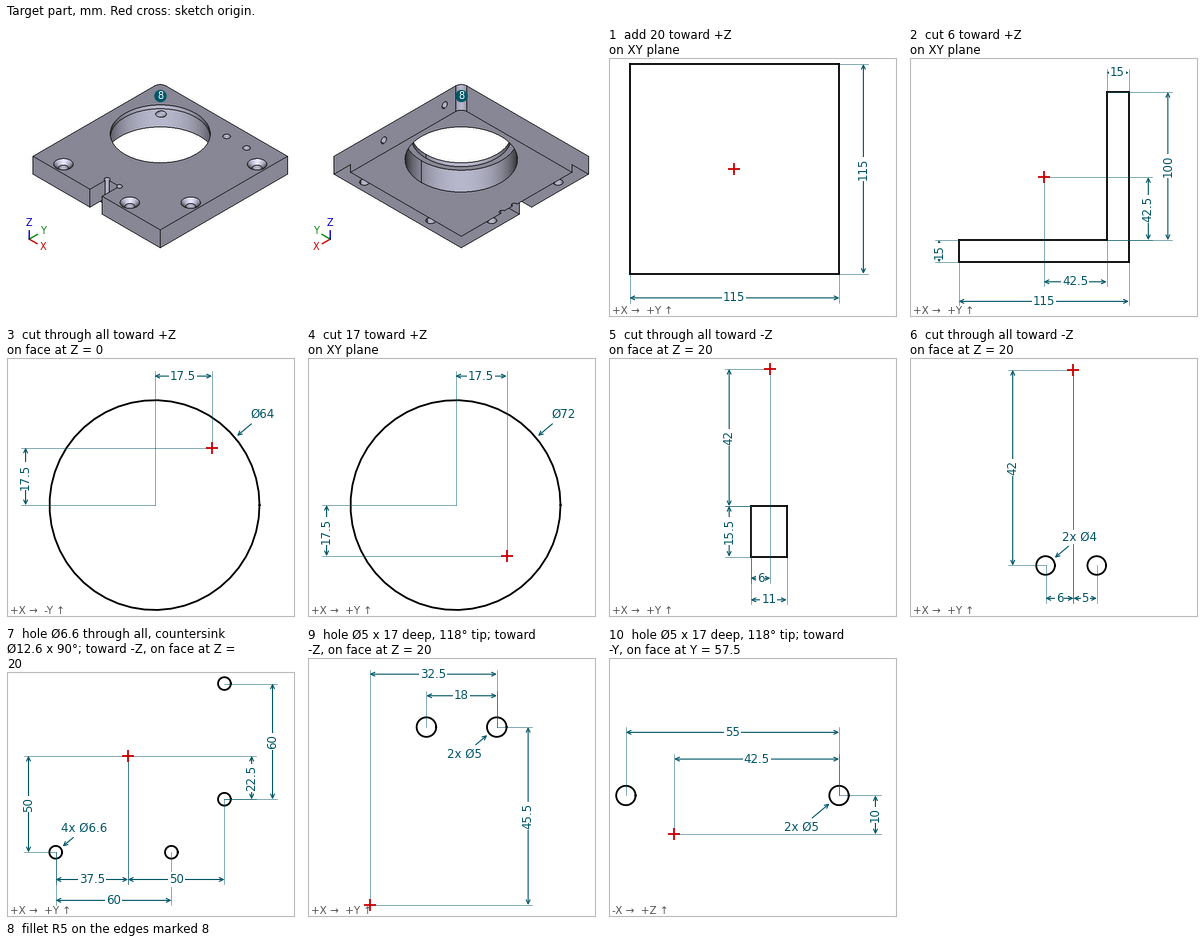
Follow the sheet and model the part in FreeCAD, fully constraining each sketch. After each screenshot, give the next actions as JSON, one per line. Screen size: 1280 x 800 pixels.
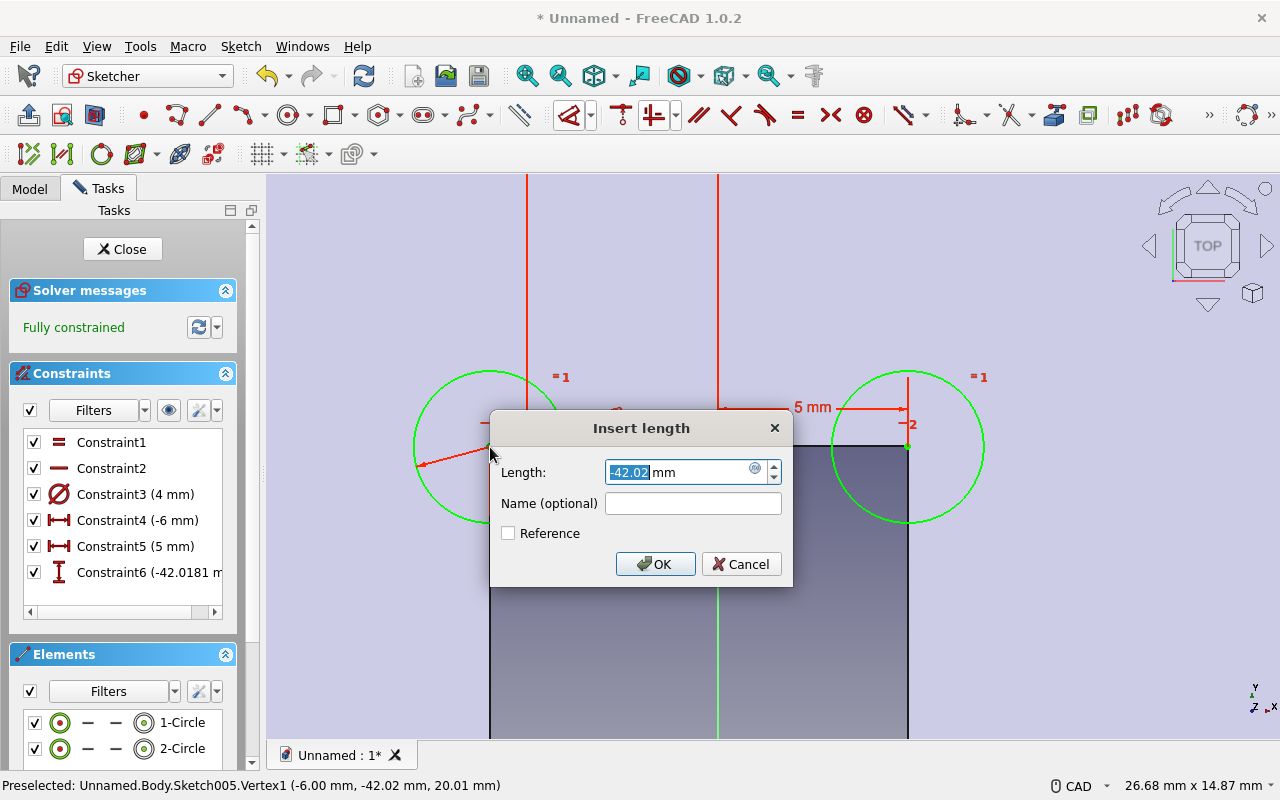
{"action": "type", "text": "-42"}
{"action": "key", "text": "Return"}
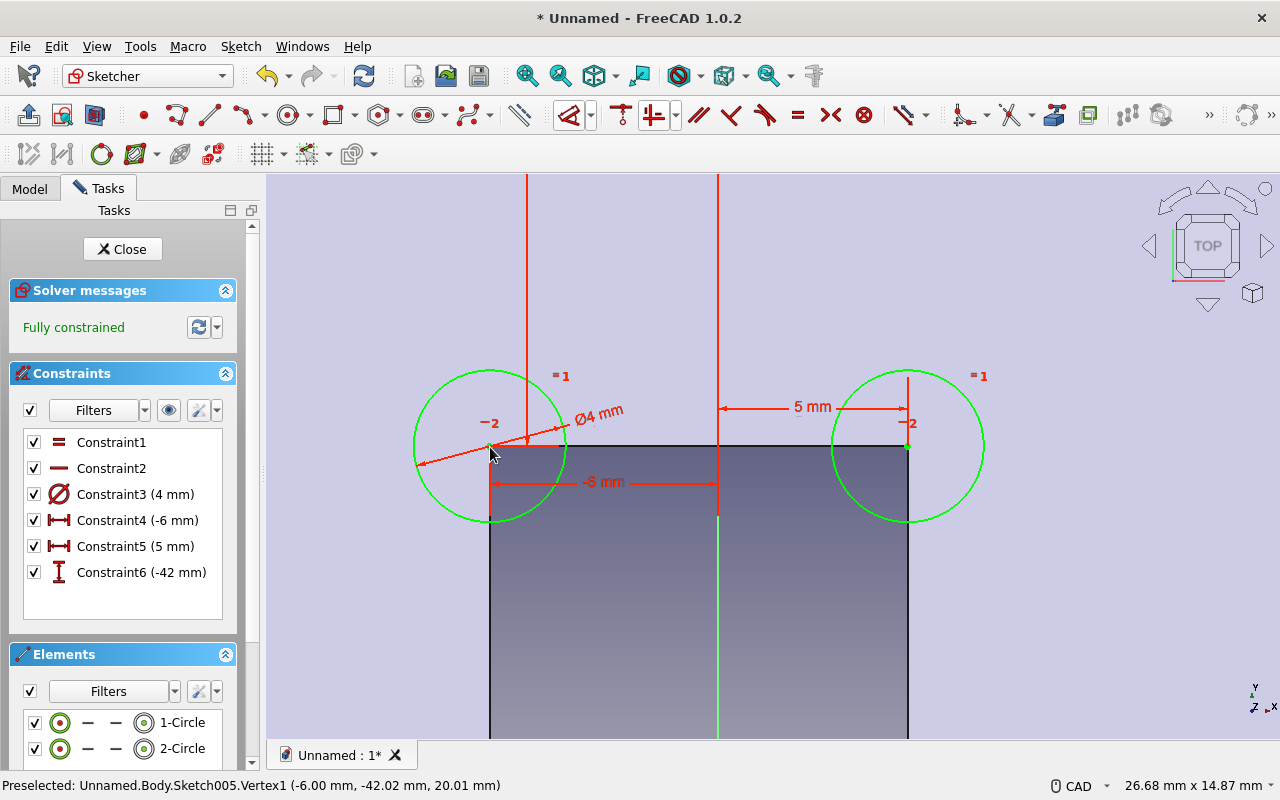
{"action": "left_click", "coordinate": [123, 249]}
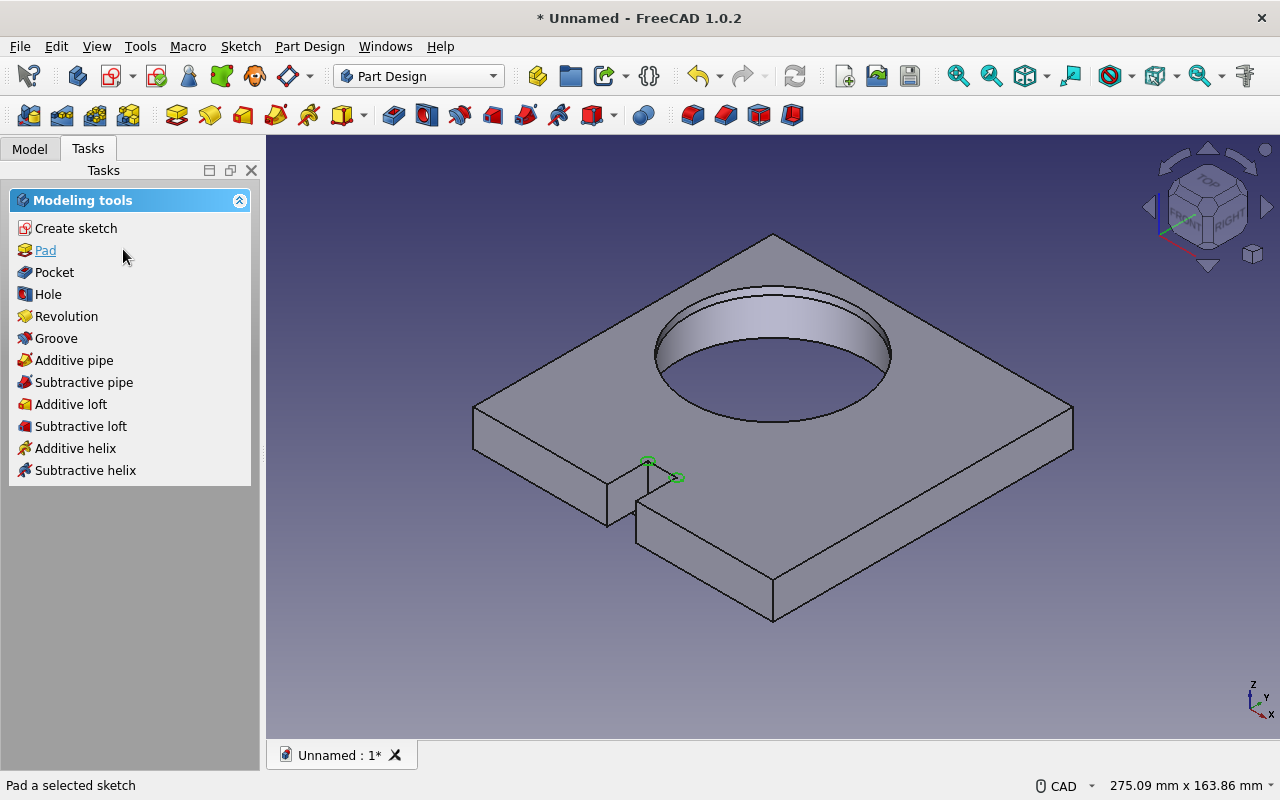
{"action": "left_click", "coordinate": [394, 116]}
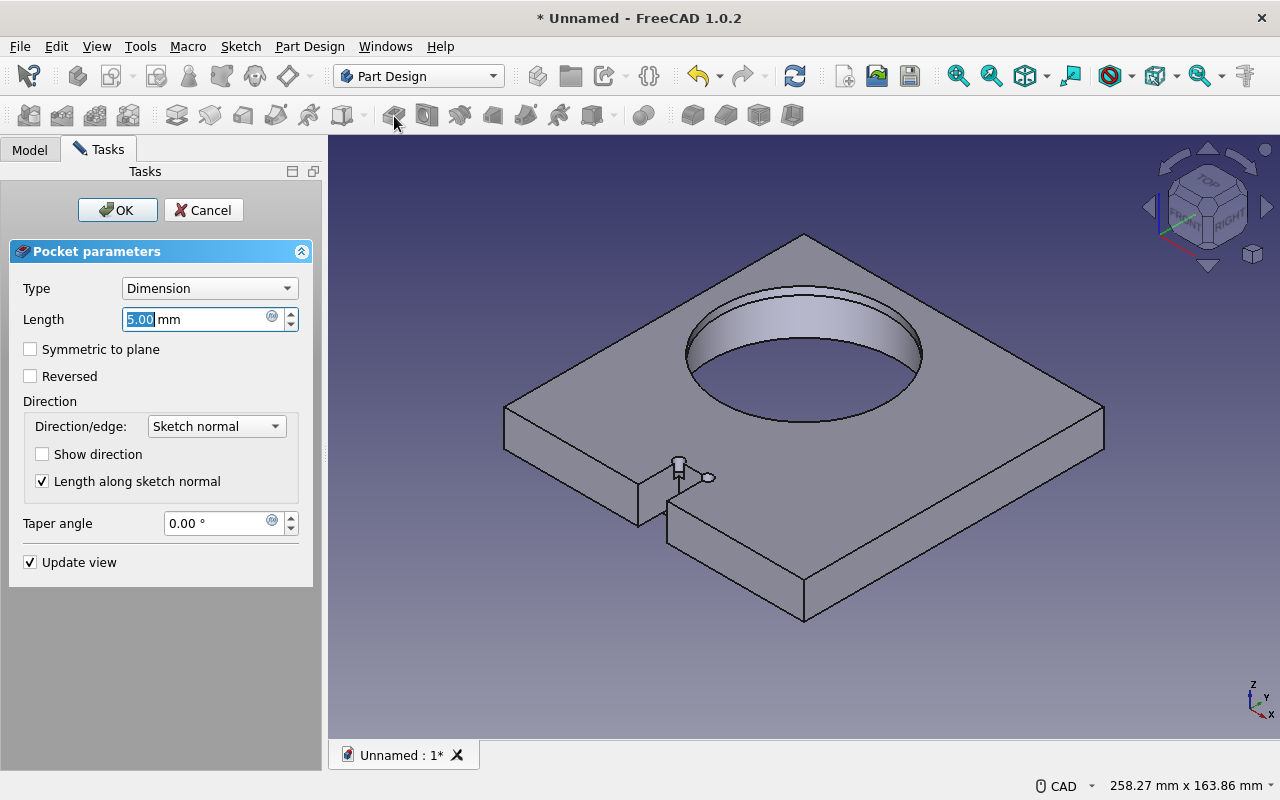
{"action": "left_click", "coordinate": [210, 288]}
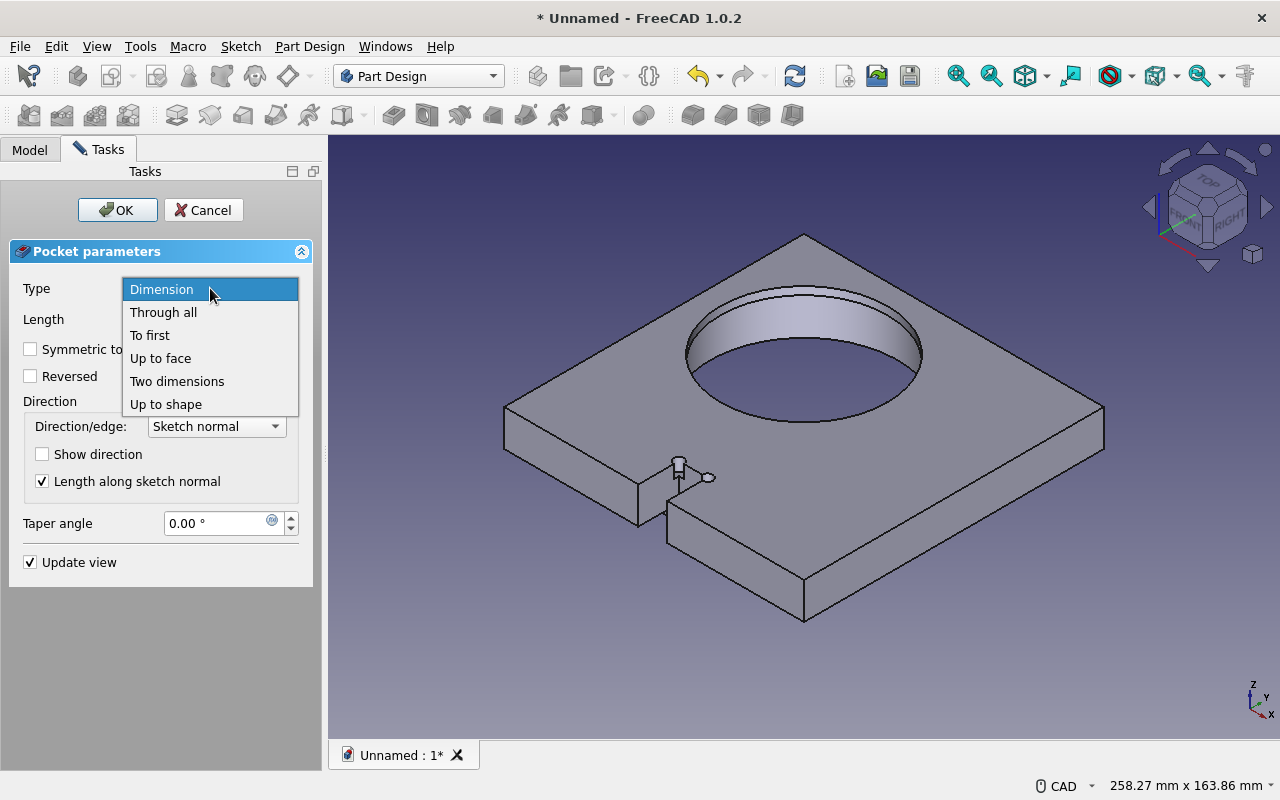
{"action": "left_click", "coordinate": [208, 312]}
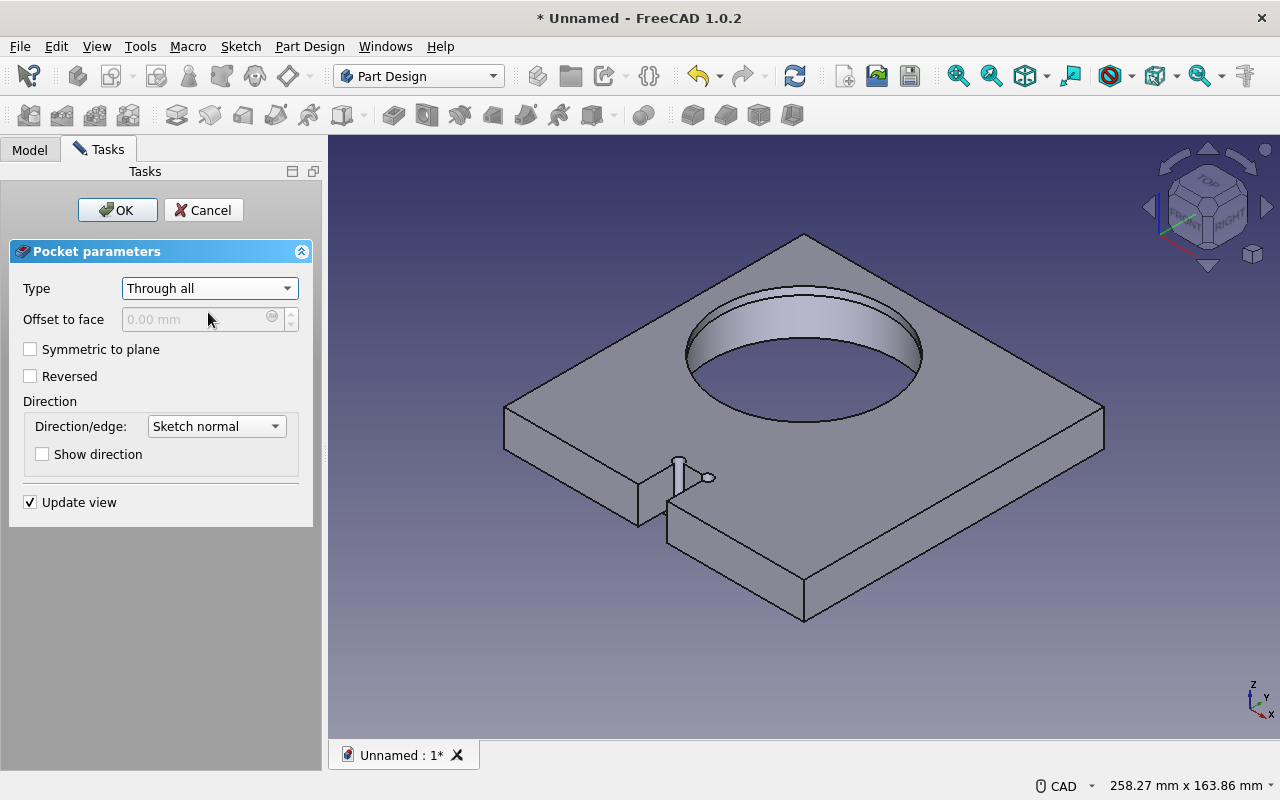
{"action": "left_click", "coordinate": [118, 210]}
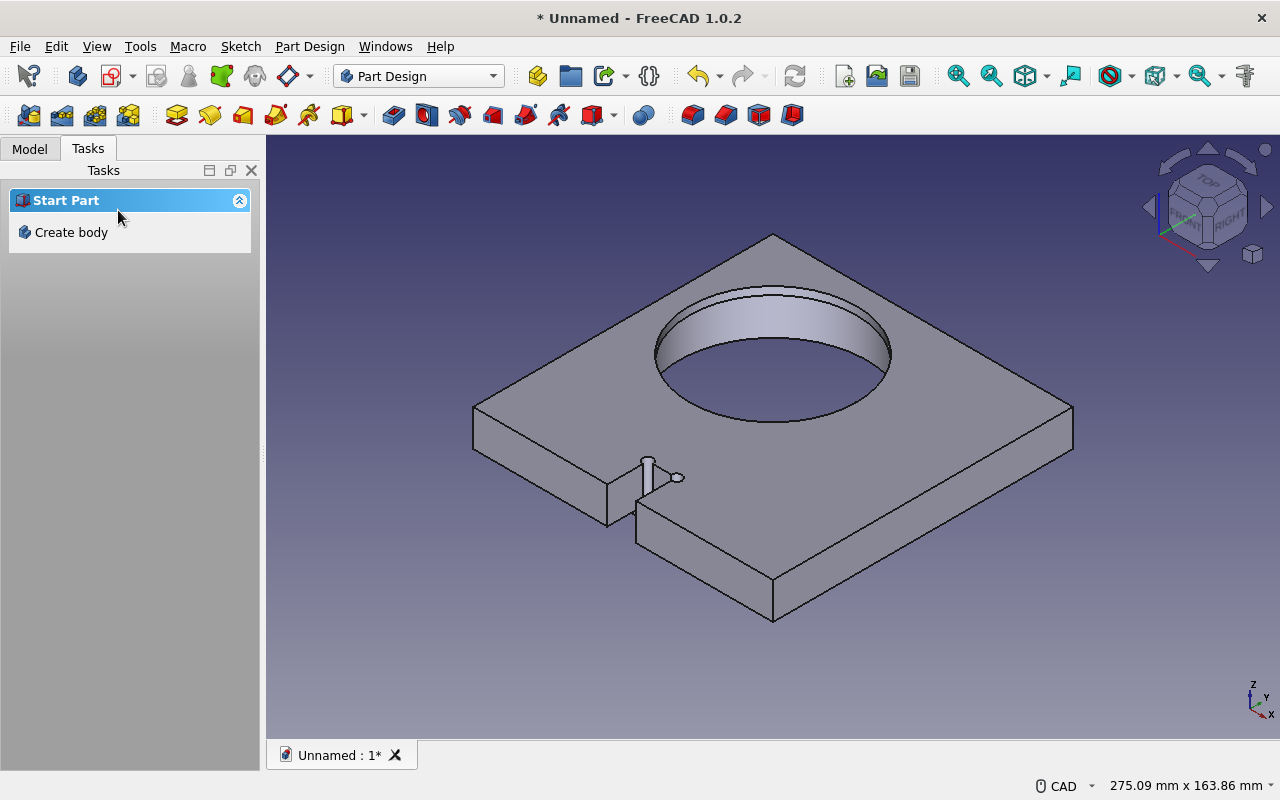
{"action": "left_click", "coordinate": [816, 480]}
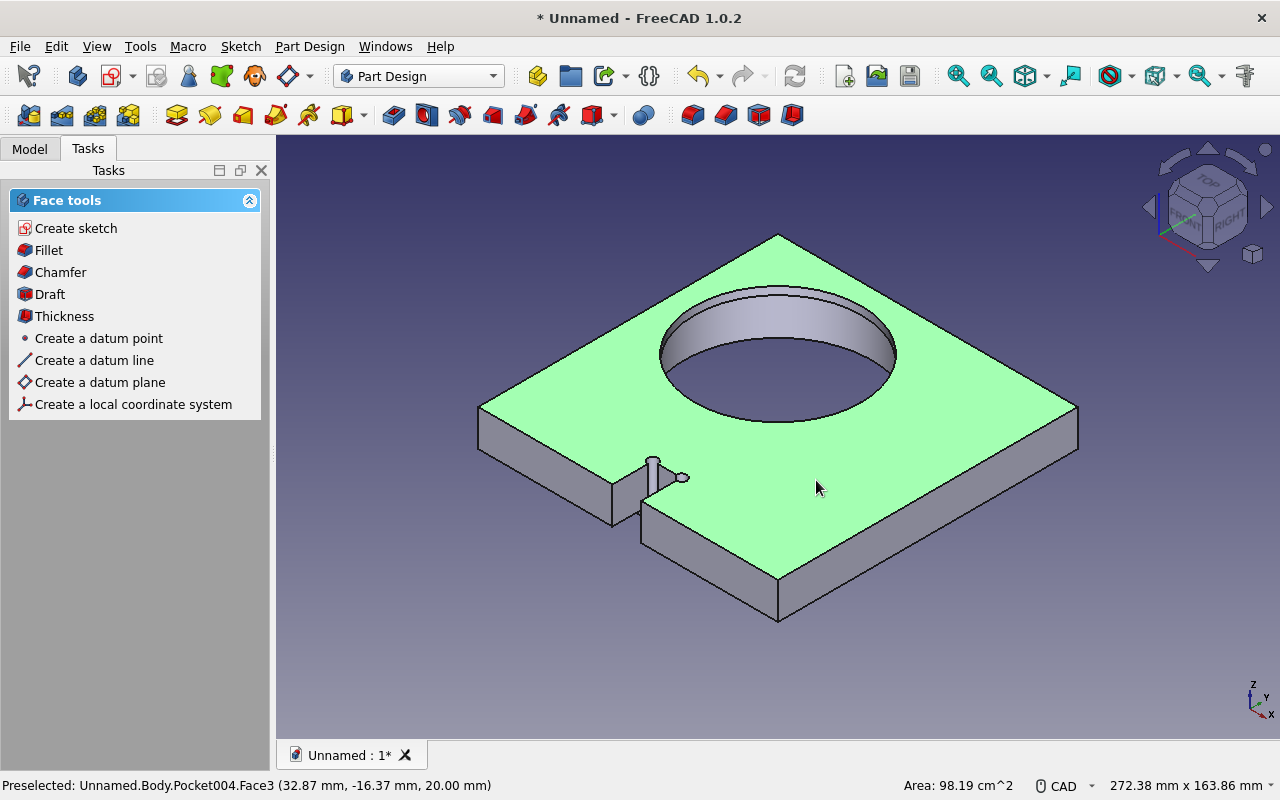
{"action": "left_click", "coordinate": [110, 76]}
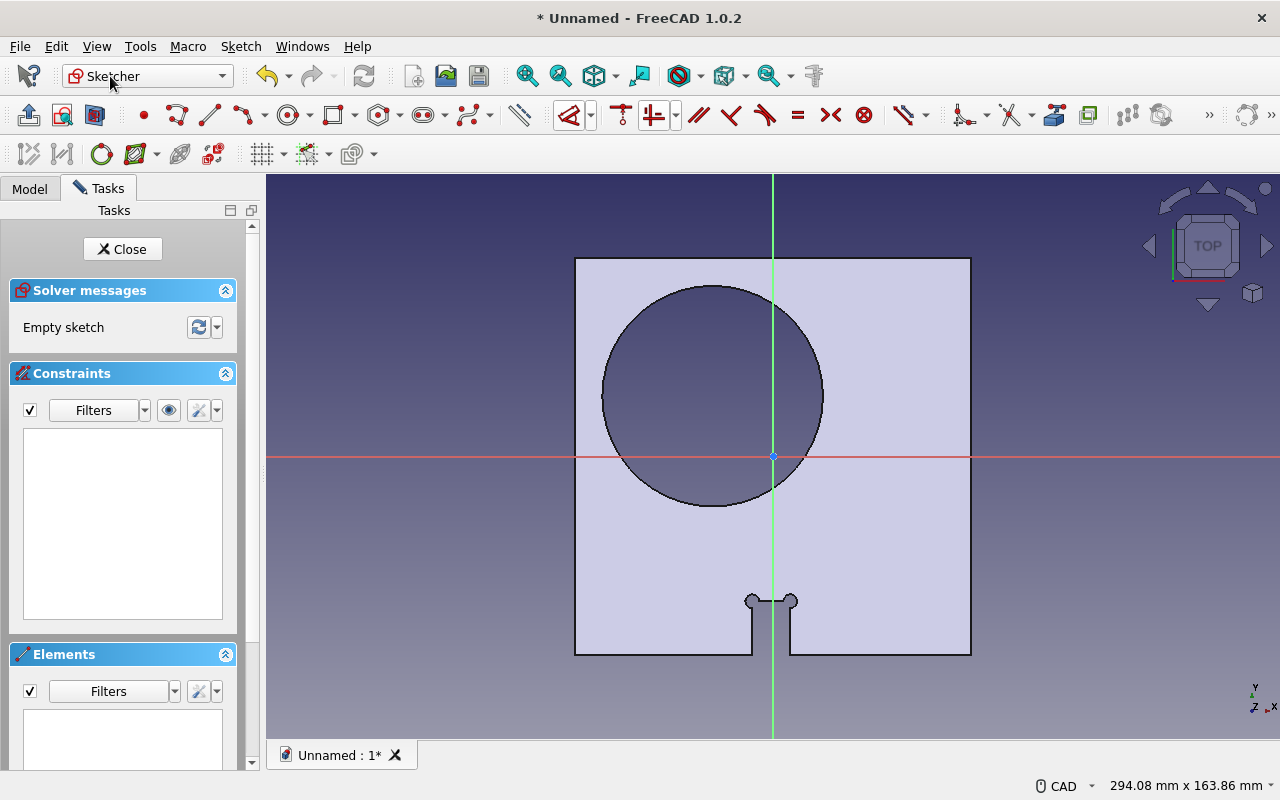
{"action": "left_click", "coordinate": [288, 116]}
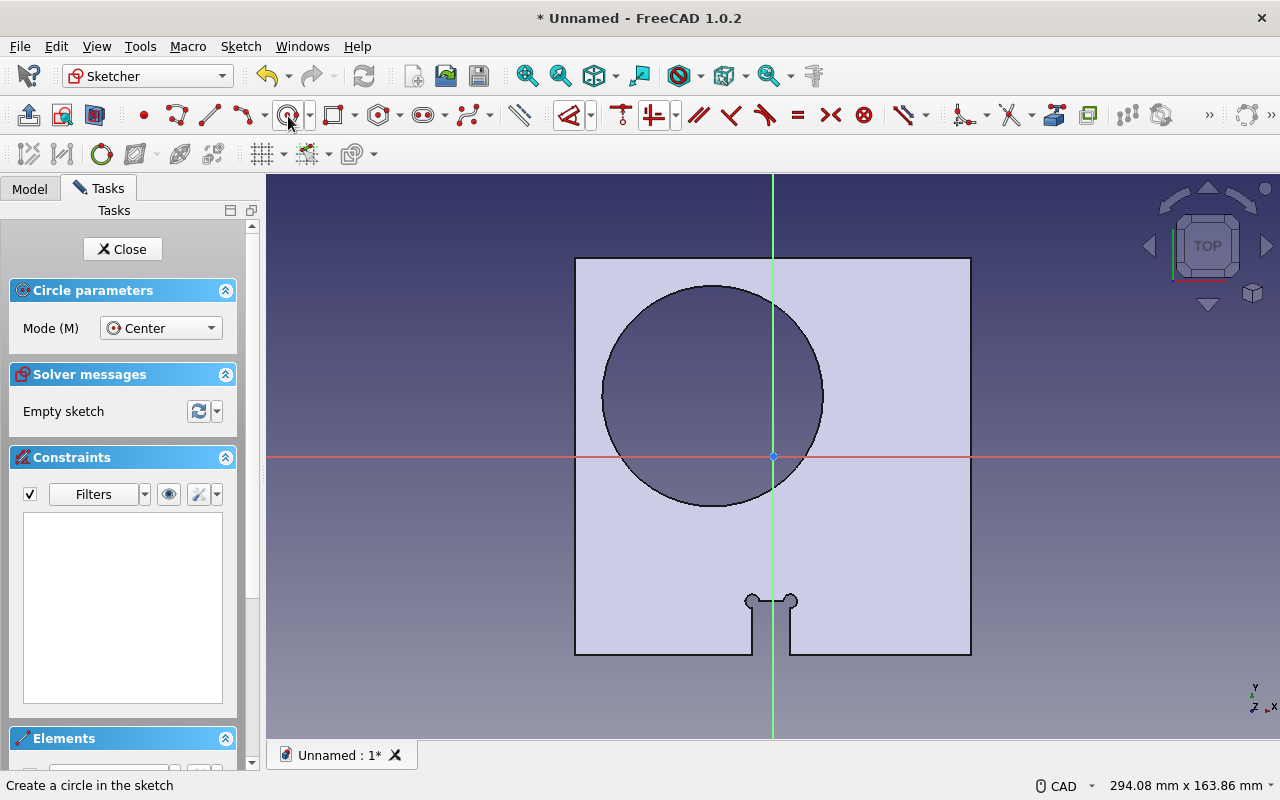
{"action": "scroll", "coordinate": [644, 629], "scroll_direction": "up", "scroll_amount": 4}